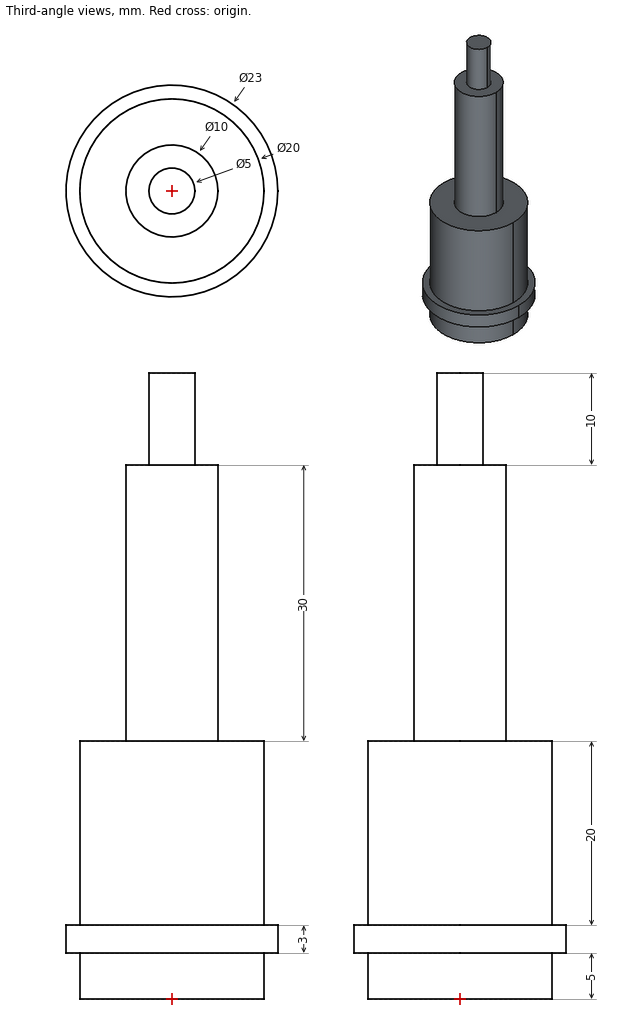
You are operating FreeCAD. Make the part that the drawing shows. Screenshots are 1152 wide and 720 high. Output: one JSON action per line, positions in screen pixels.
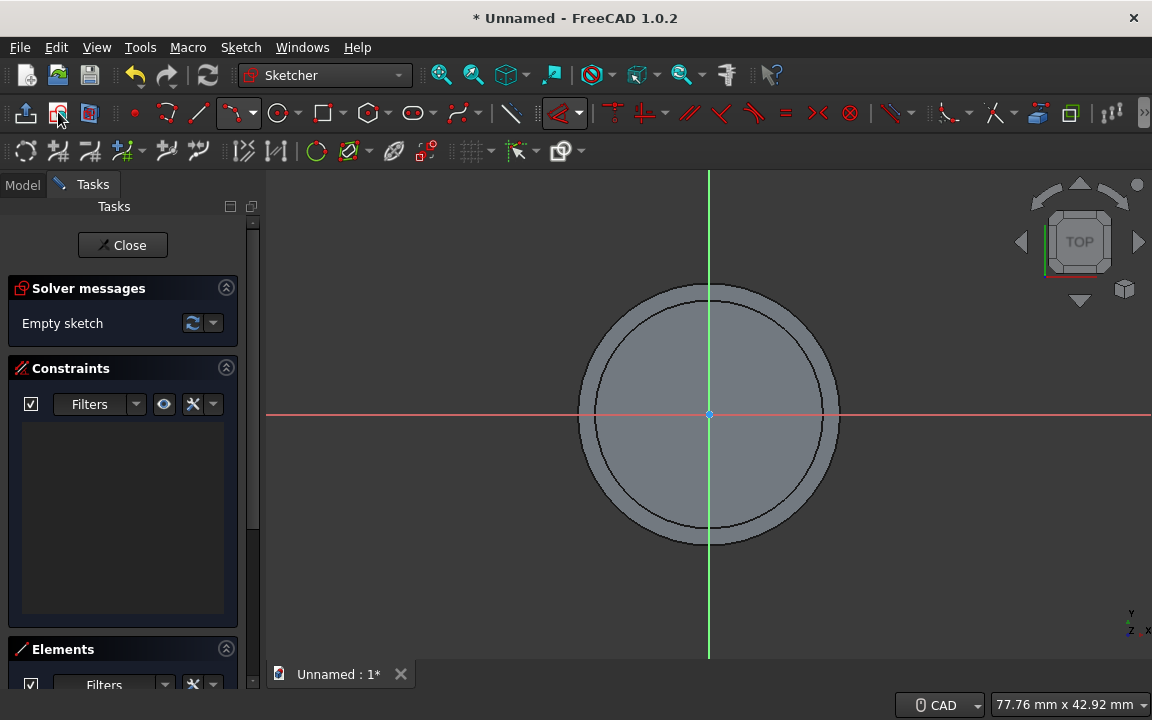
{"action": "scroll", "coordinate": [749, 415], "scroll_direction": "up", "scroll_amount": 5}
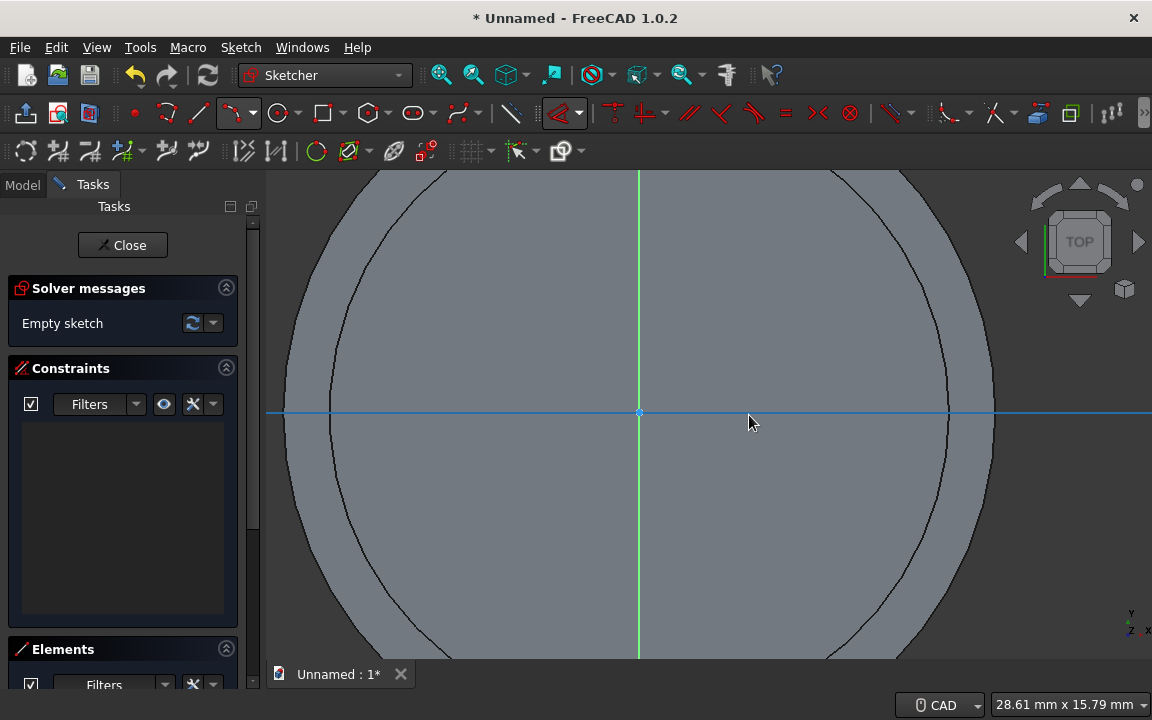
{"action": "left_click", "coordinate": [278, 114]}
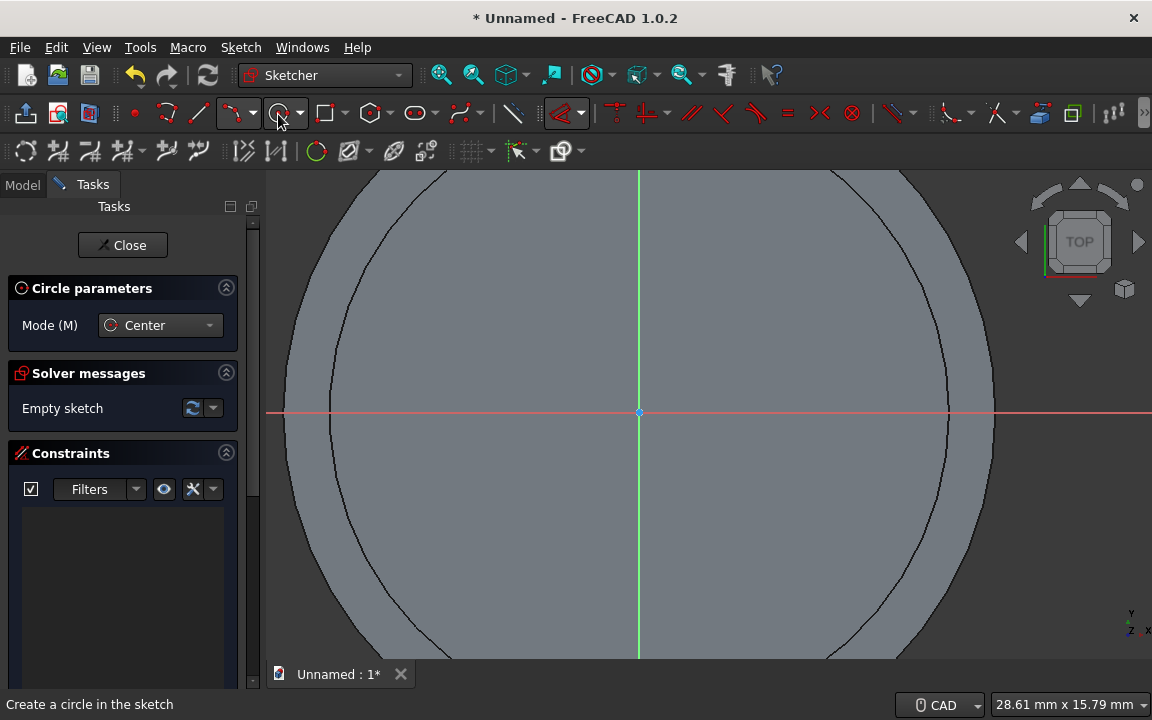
{"action": "left_click", "coordinate": [639, 413]}
{"action": "mouse_move", "coordinate": [749, 303]}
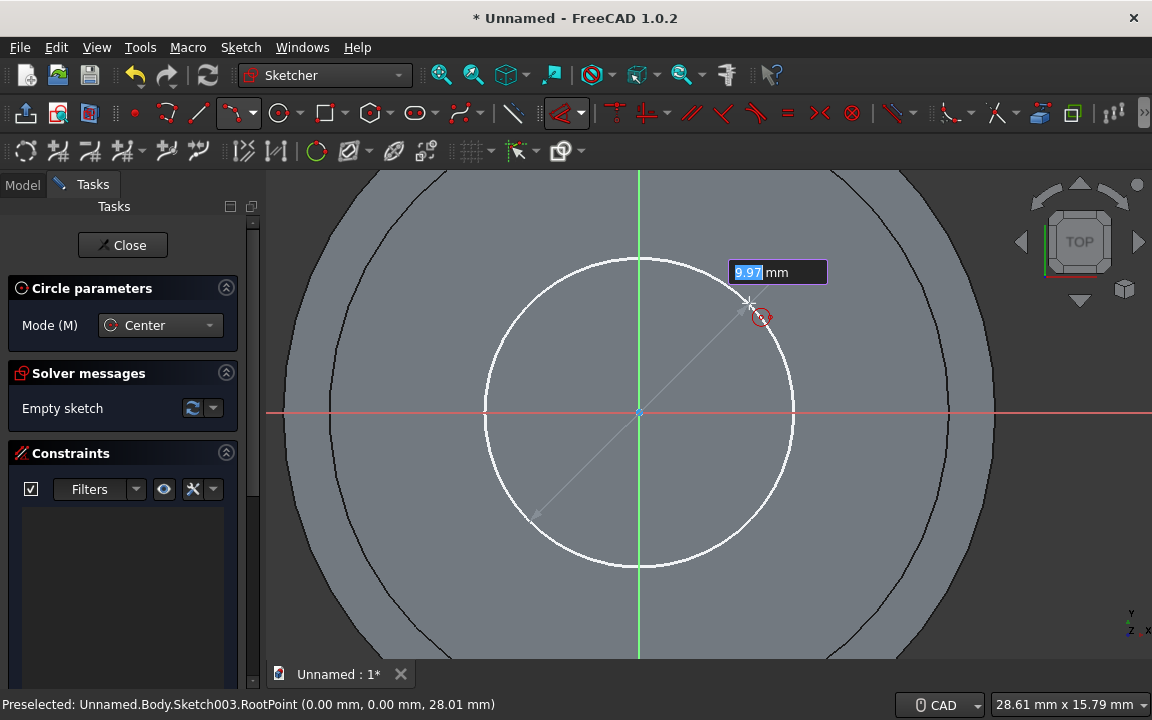
{"action": "type", "text": "10"}
{"action": "key", "text": "Return"}
{"action": "key", "text": "Escape"}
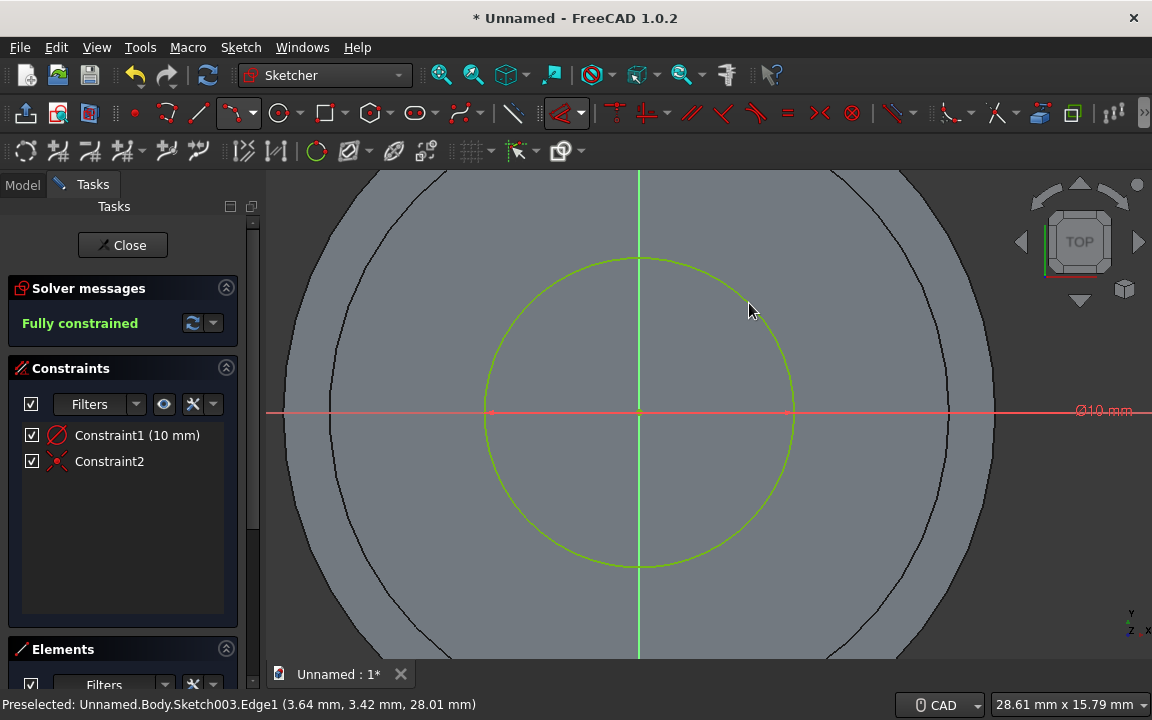
{"action": "left_click", "coordinate": [123, 245]}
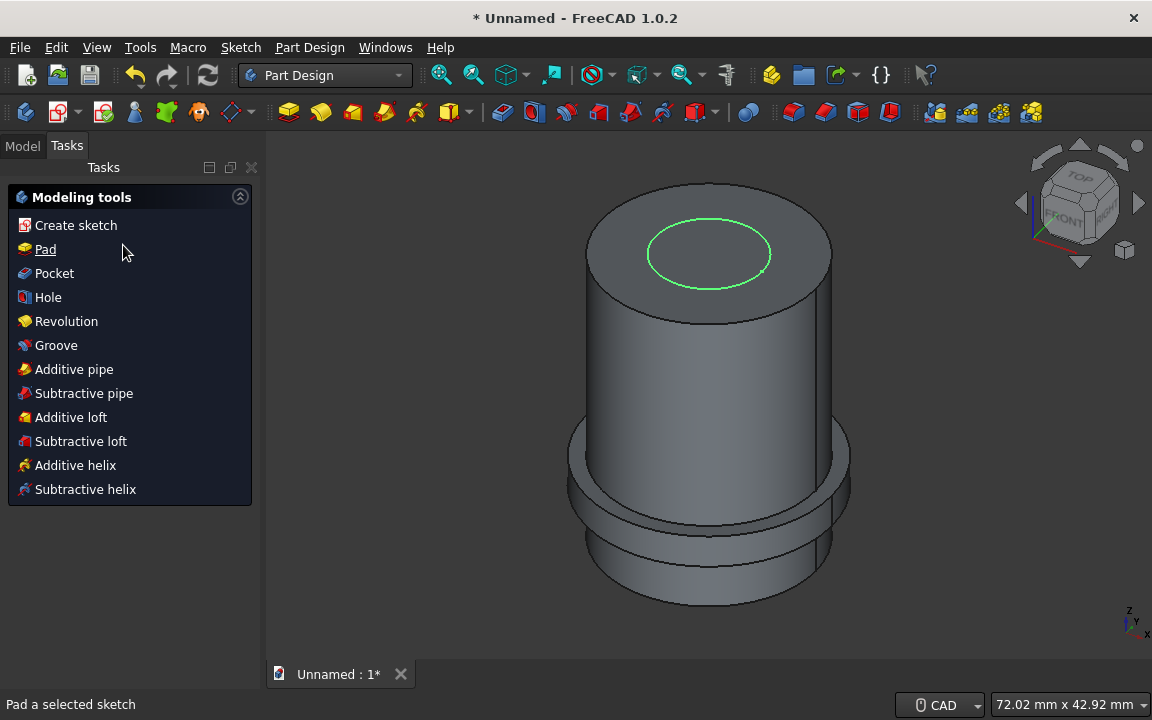
{"action": "left_click", "coordinate": [290, 112]}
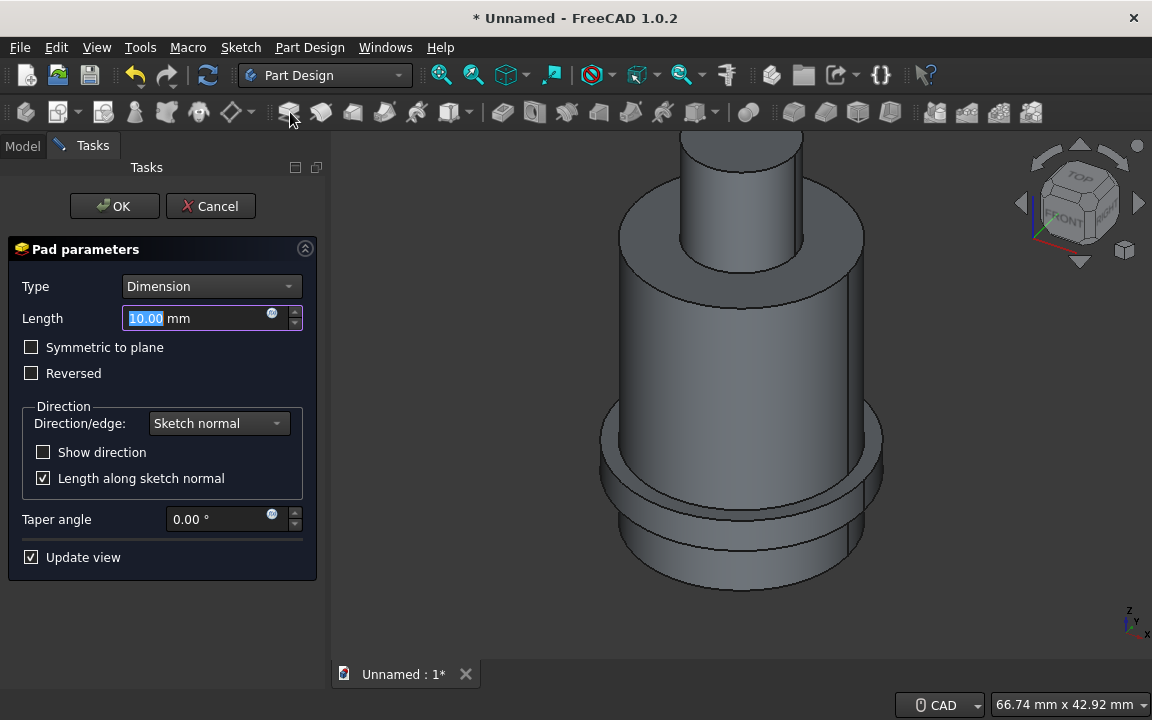
{"action": "type", "text": "30"}
{"action": "key", "text": "Tab"}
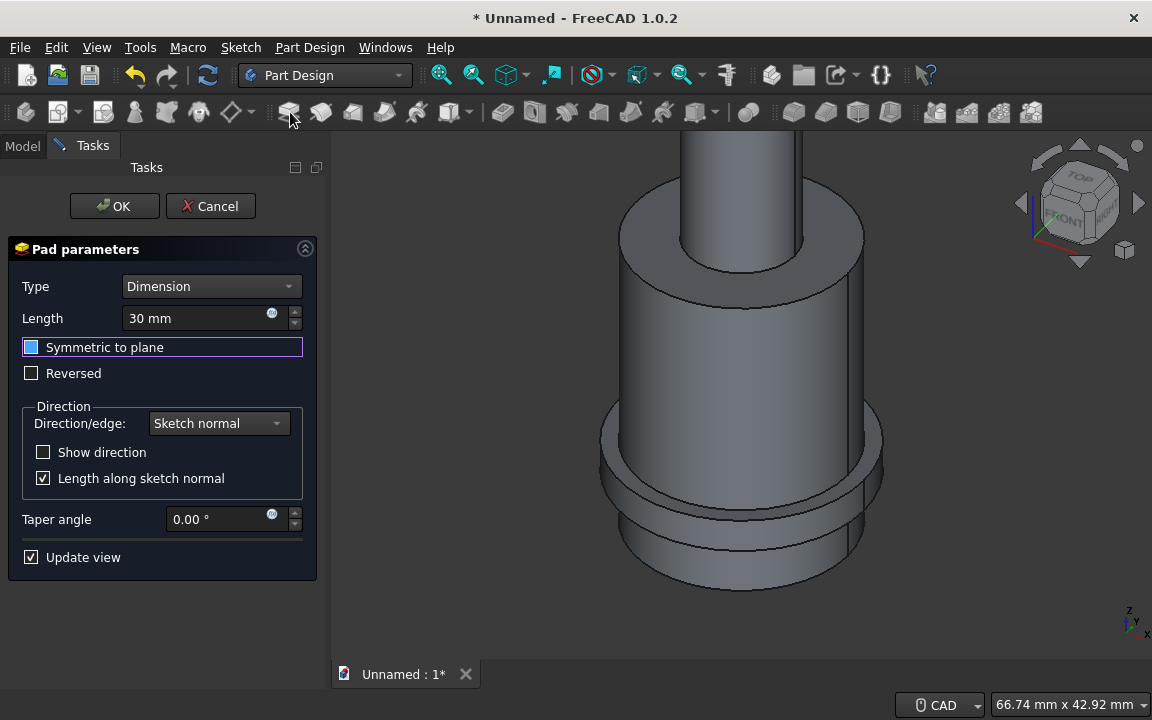
{"action": "left_click", "coordinate": [115, 206]}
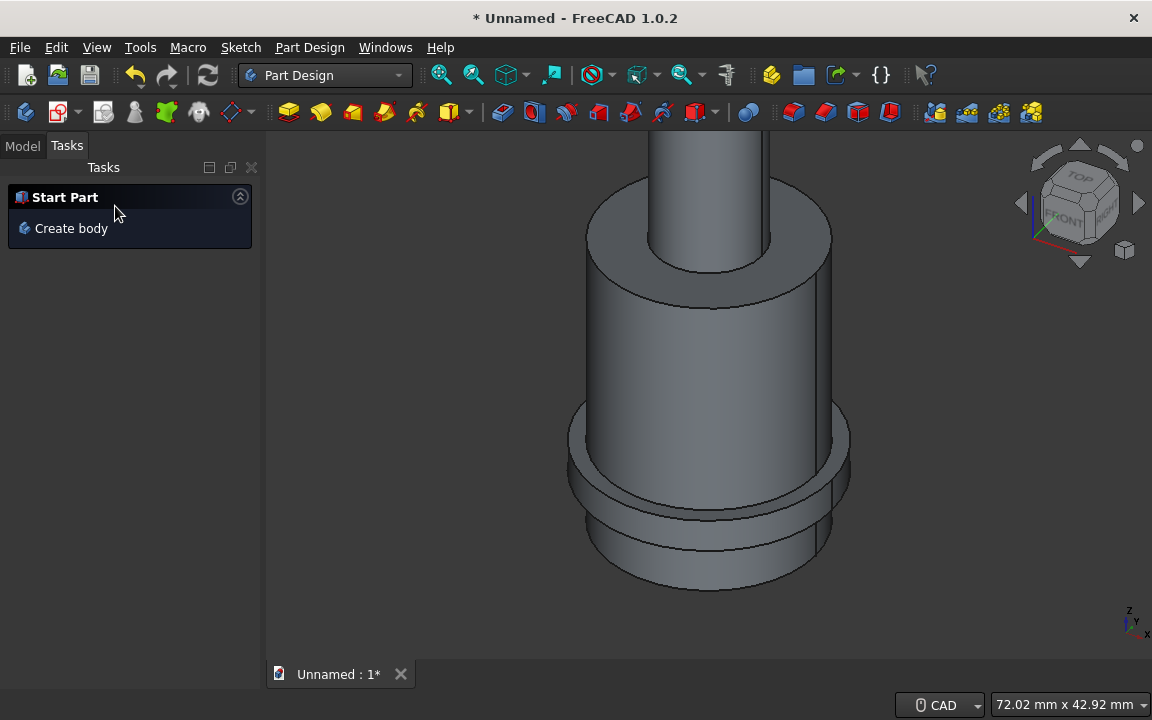
{"action": "left_click", "coordinate": [442, 76]}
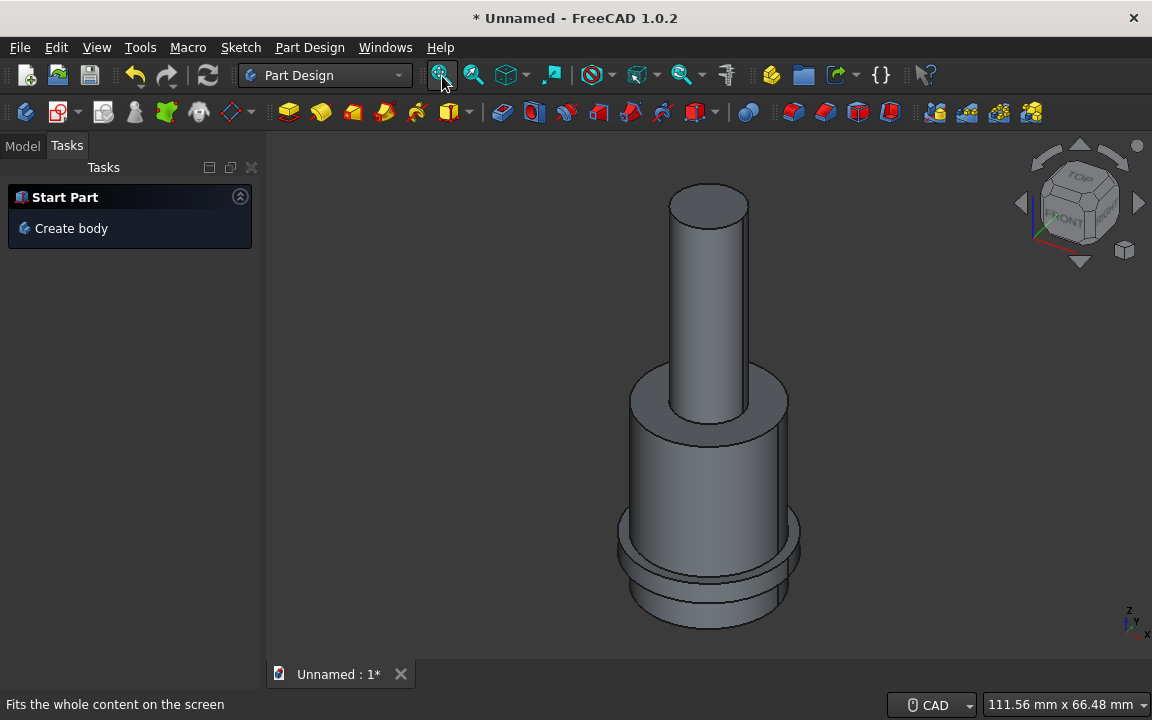
{"action": "left_click", "coordinate": [709, 205]}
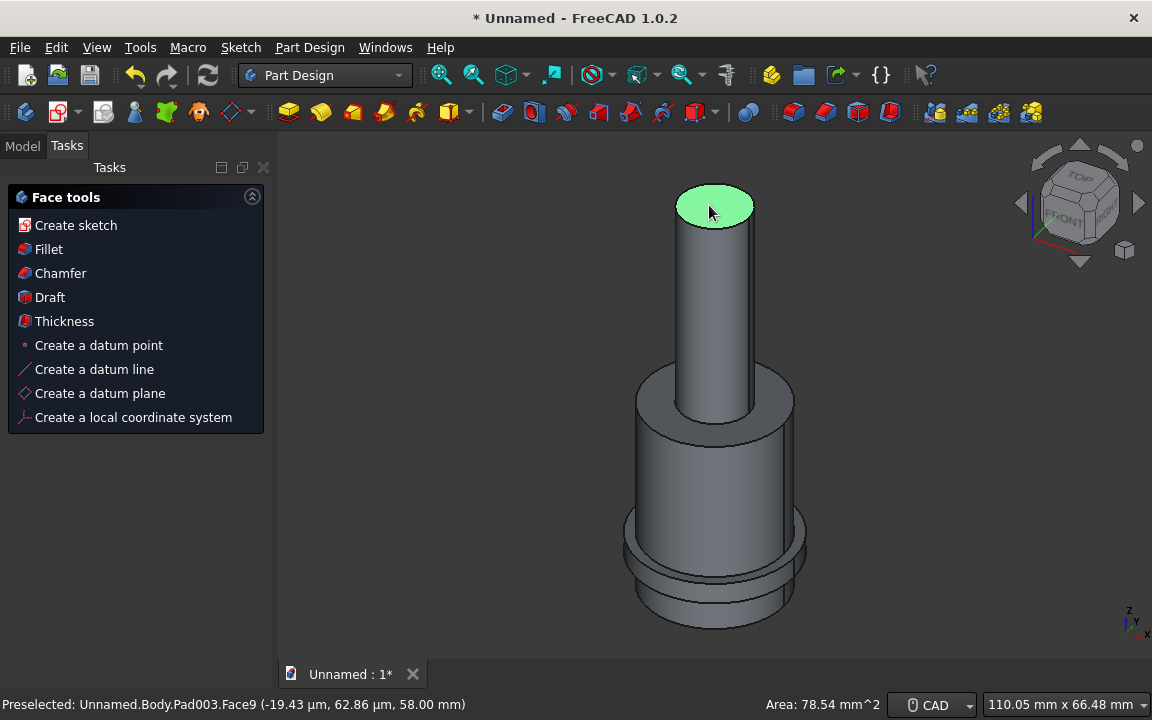
{"action": "left_click", "coordinate": [58, 112]}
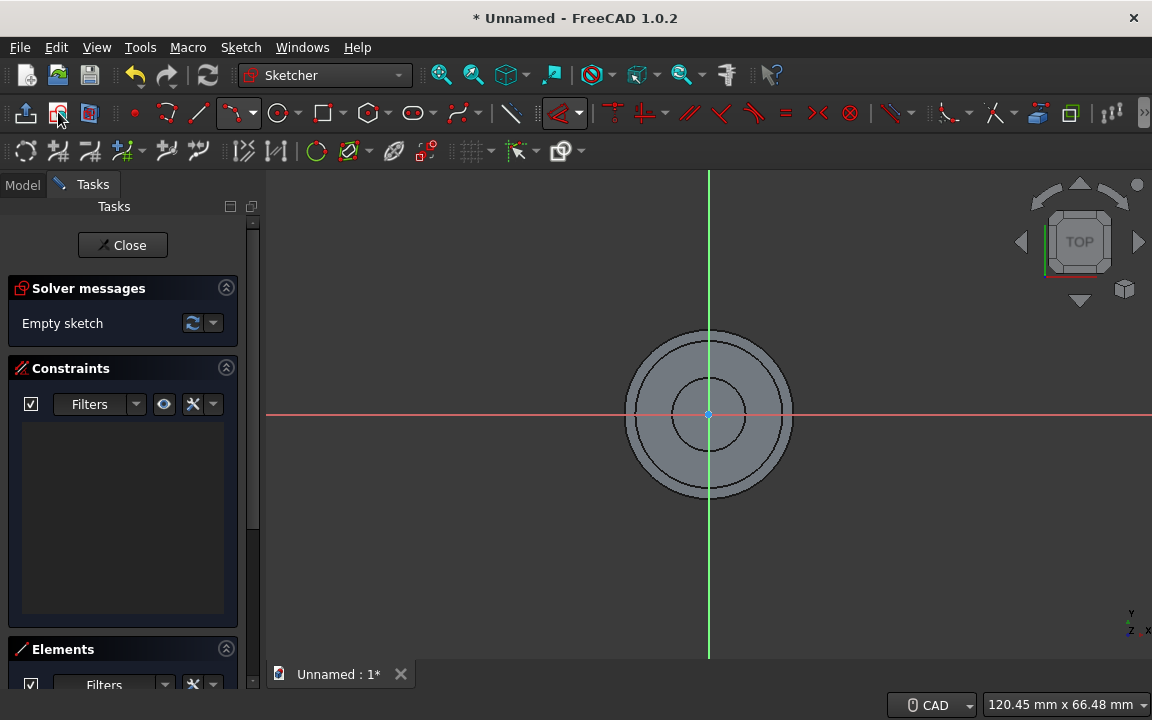
{"action": "scroll", "coordinate": [717, 414], "scroll_direction": "up", "scroll_amount": 11}